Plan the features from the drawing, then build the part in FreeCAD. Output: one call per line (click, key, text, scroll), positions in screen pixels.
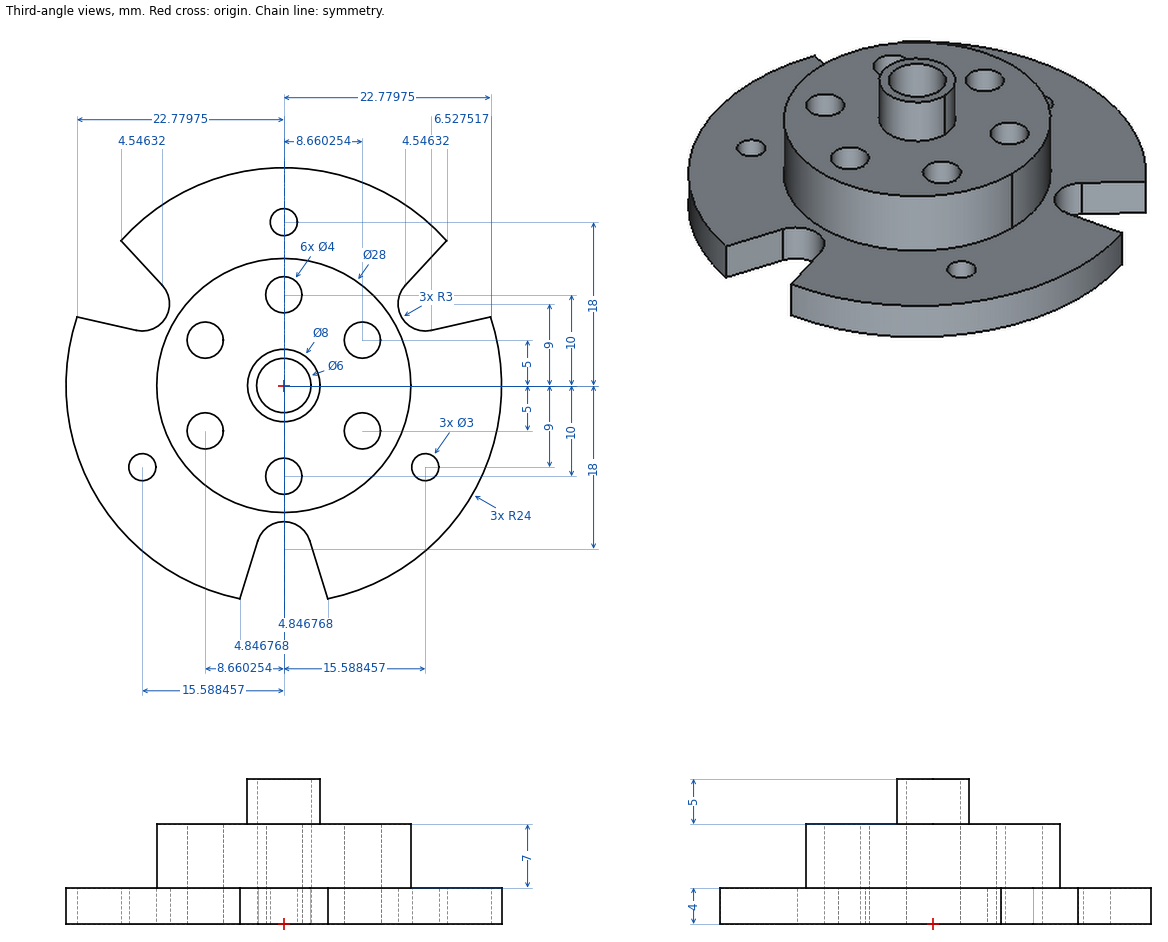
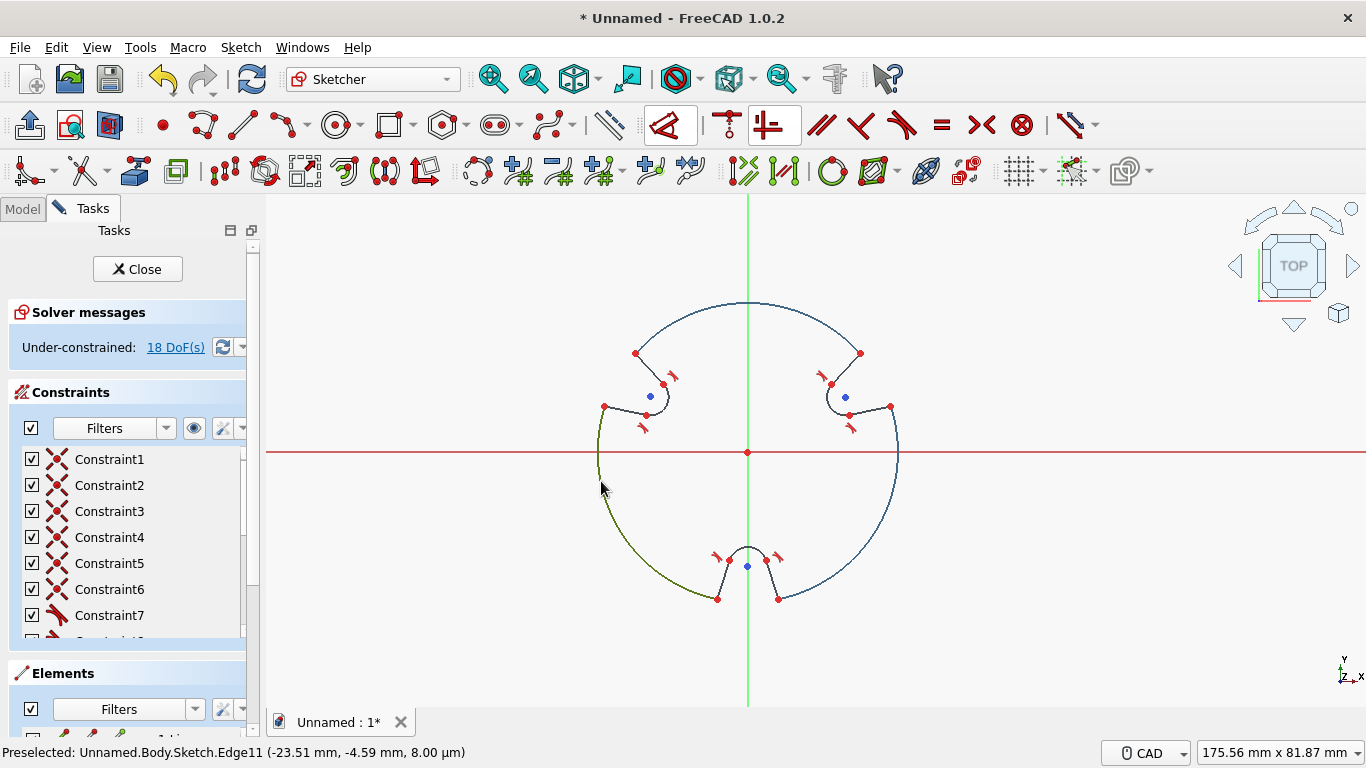
key(e)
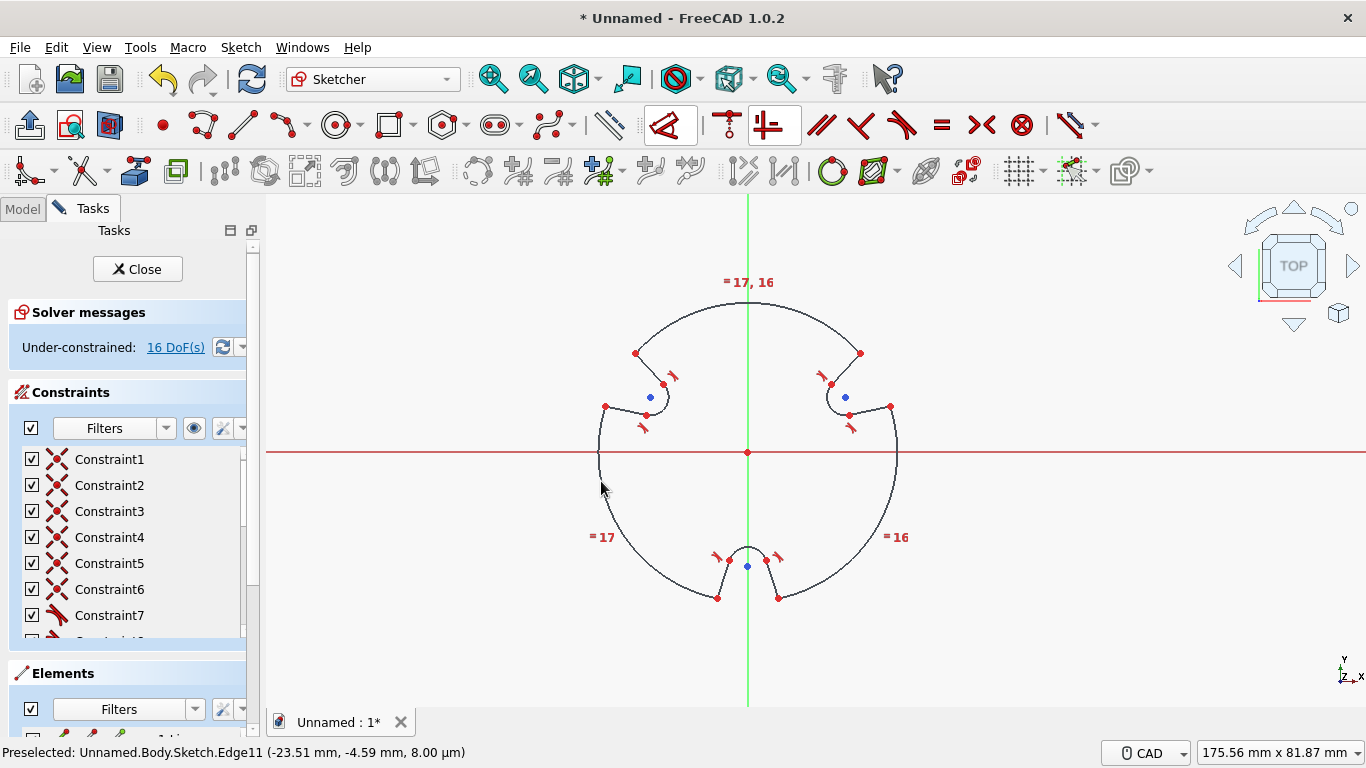
click(827, 397)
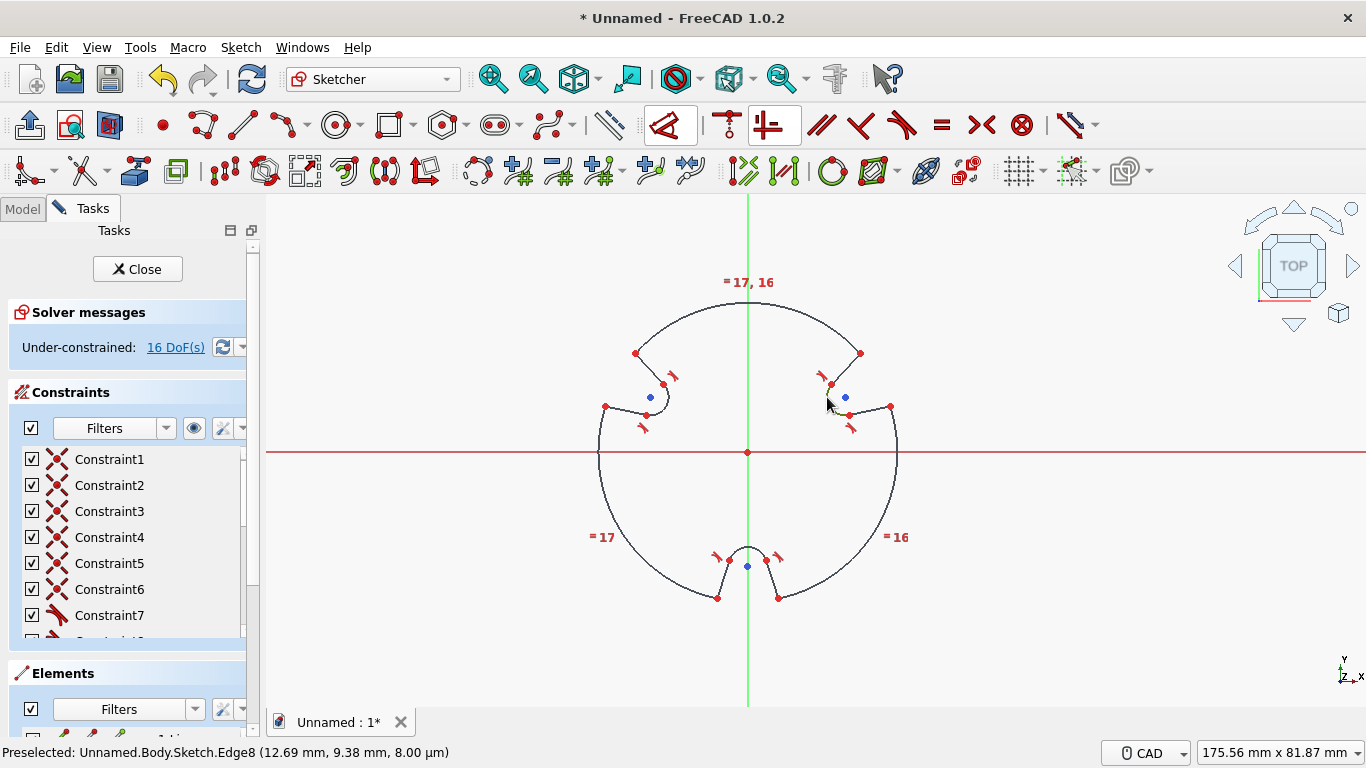
click(660, 413)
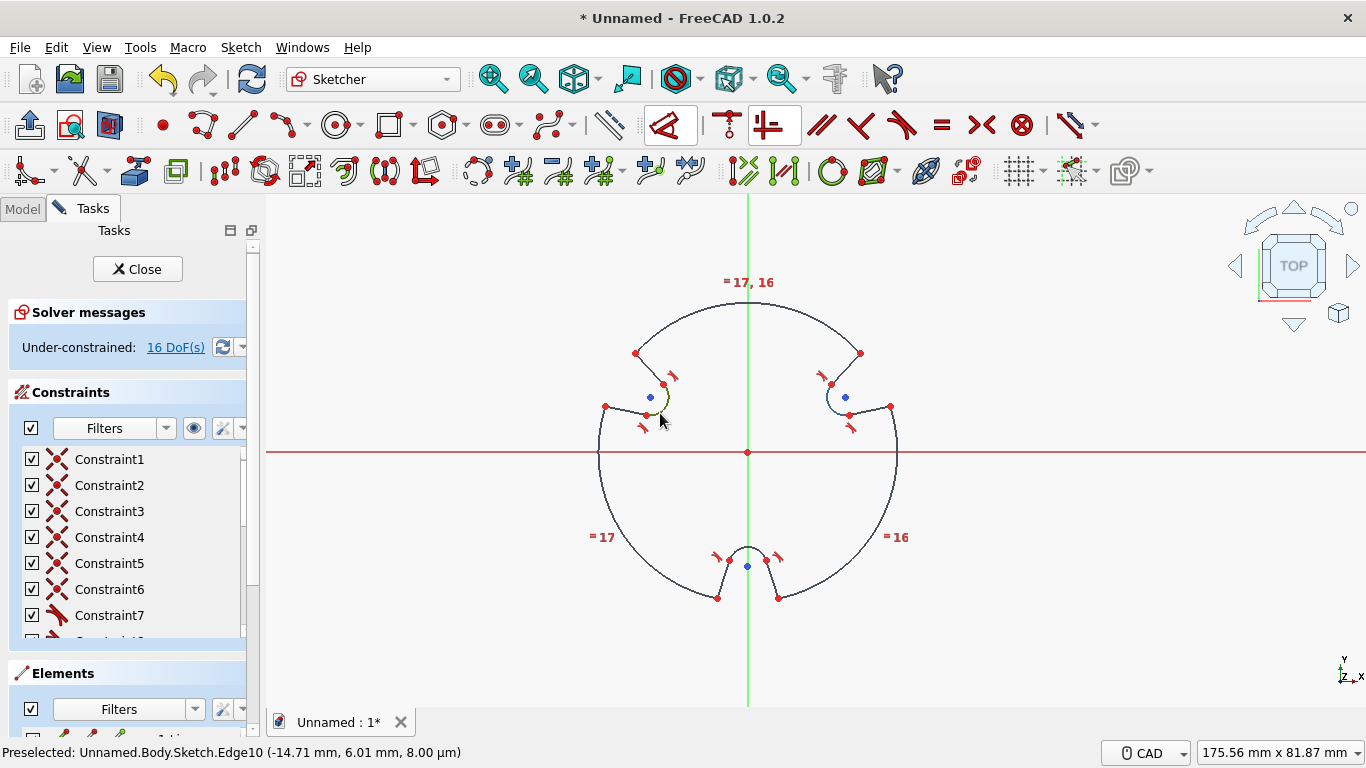
scroll(757, 549, up, 2)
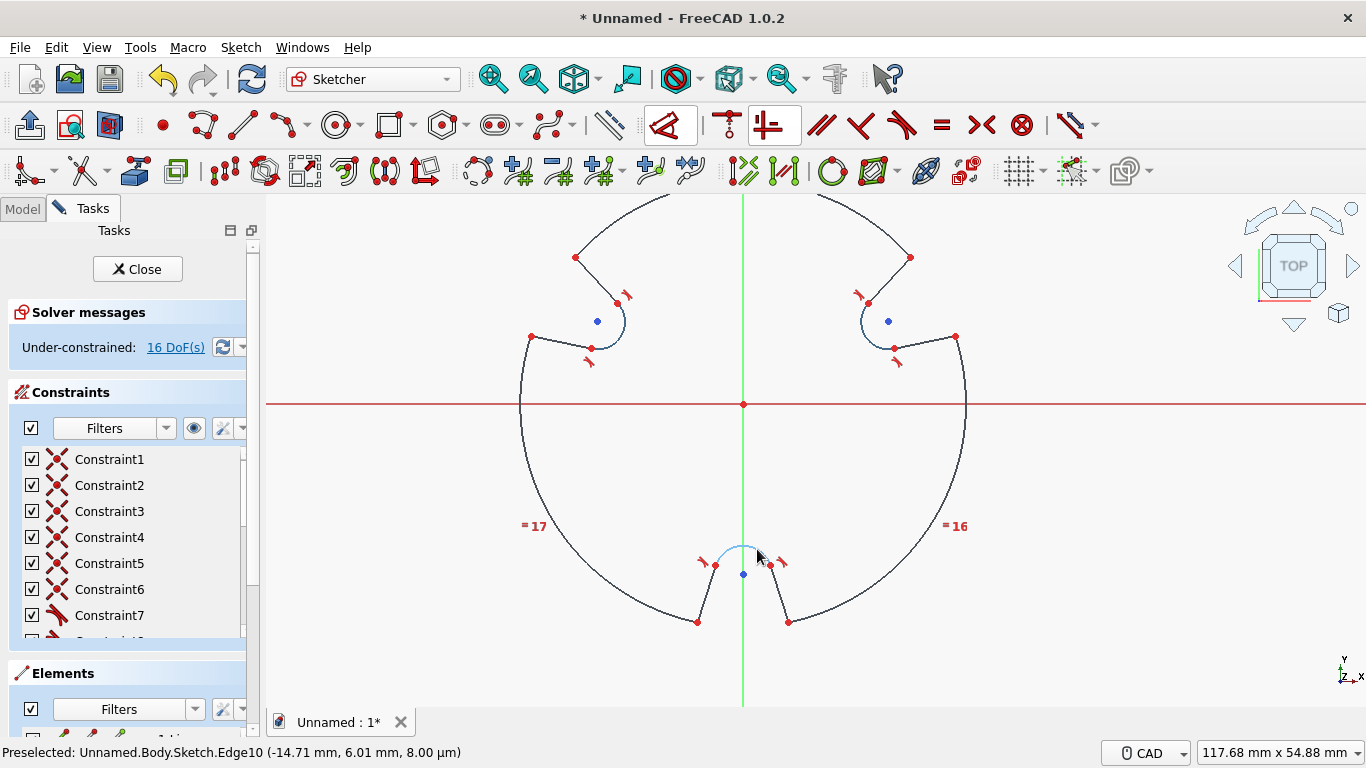
click(757, 549)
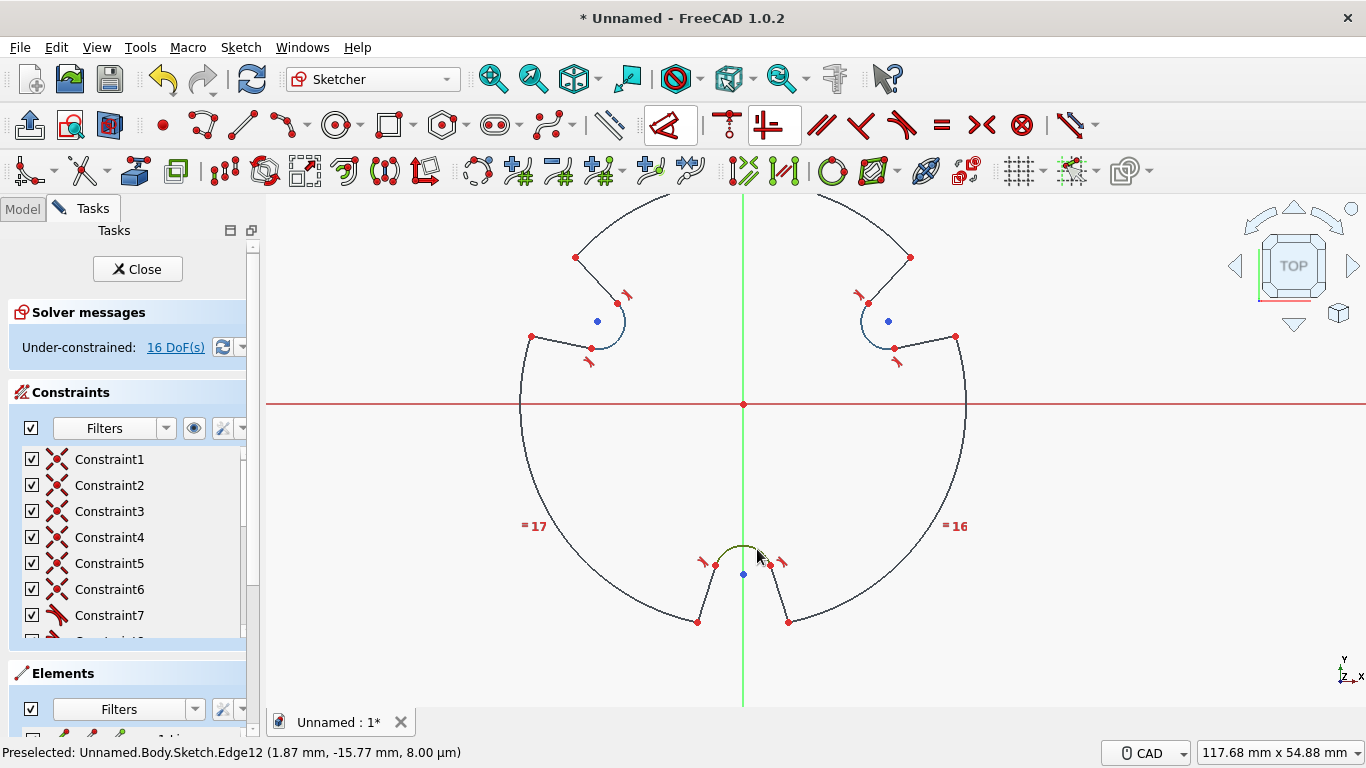
key(e)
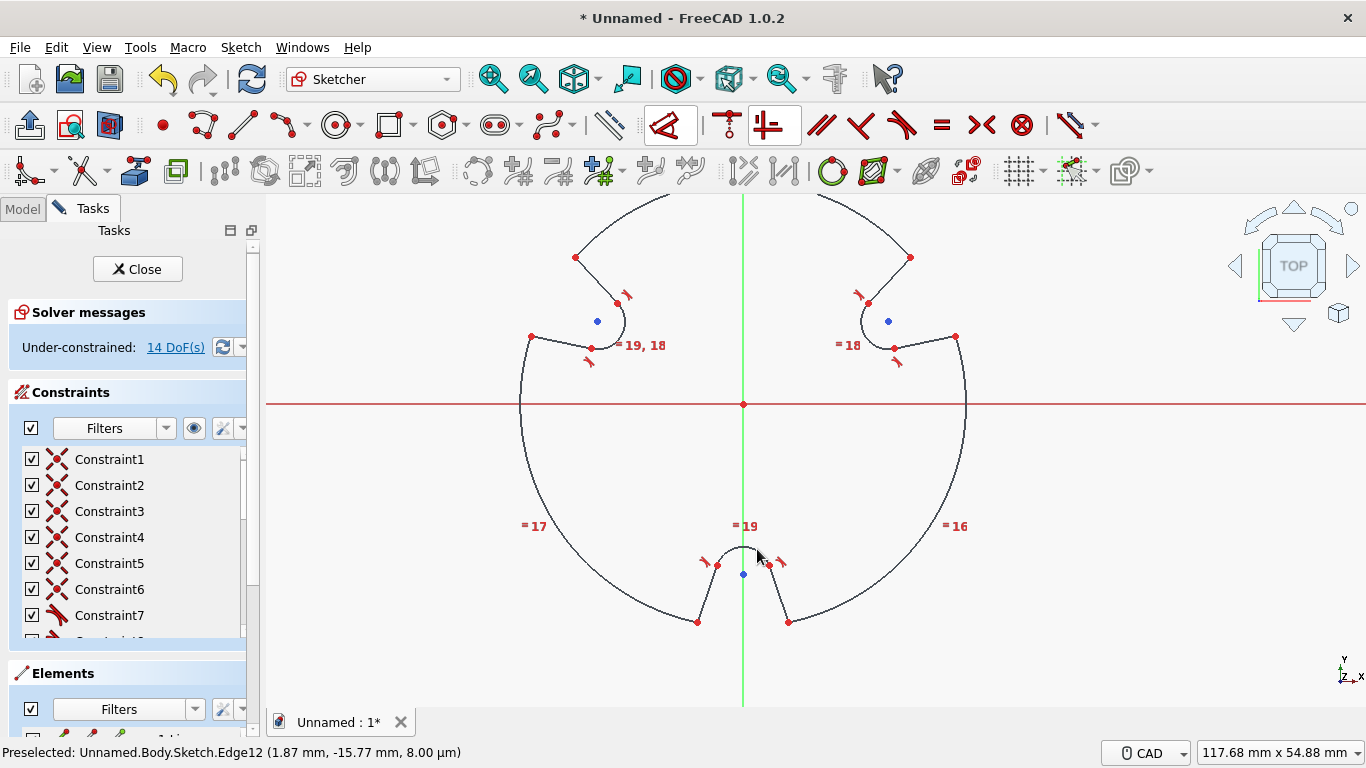
click(743, 574)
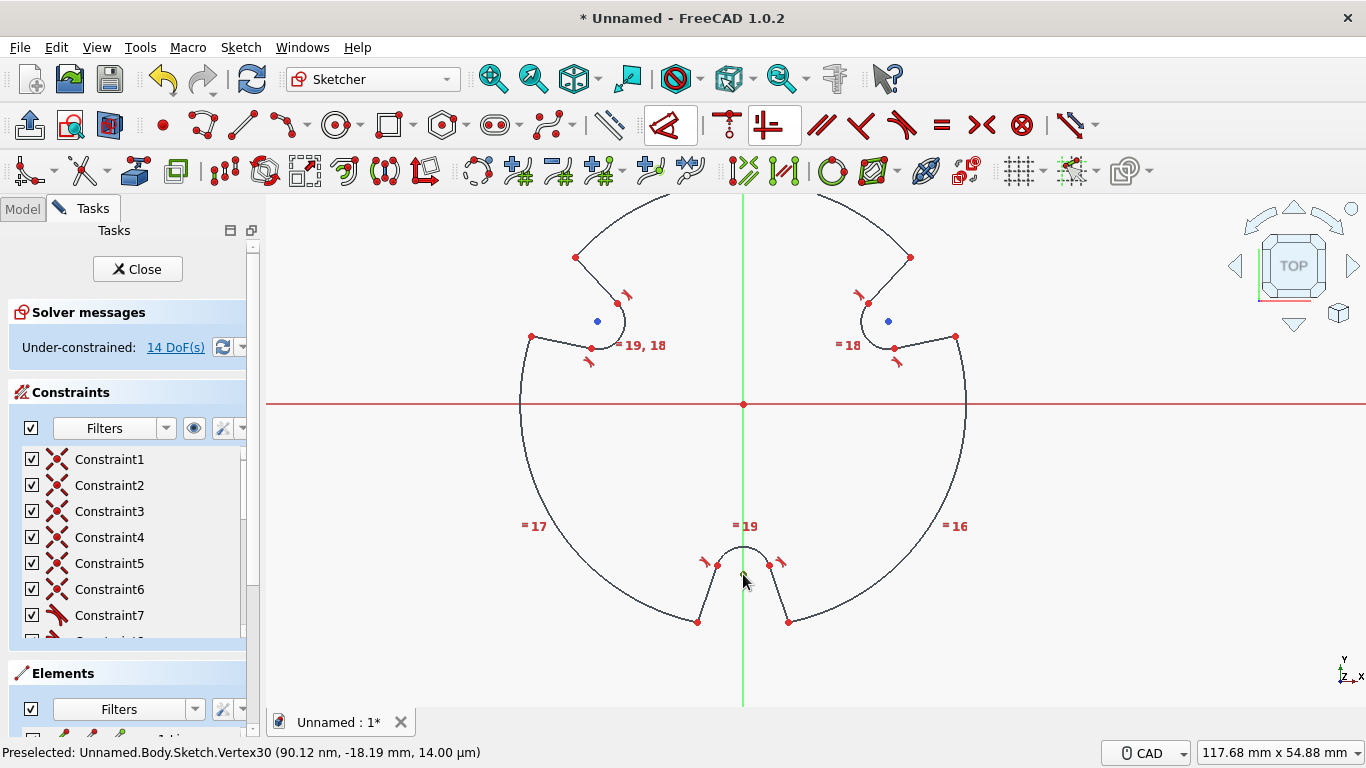
click(743, 646)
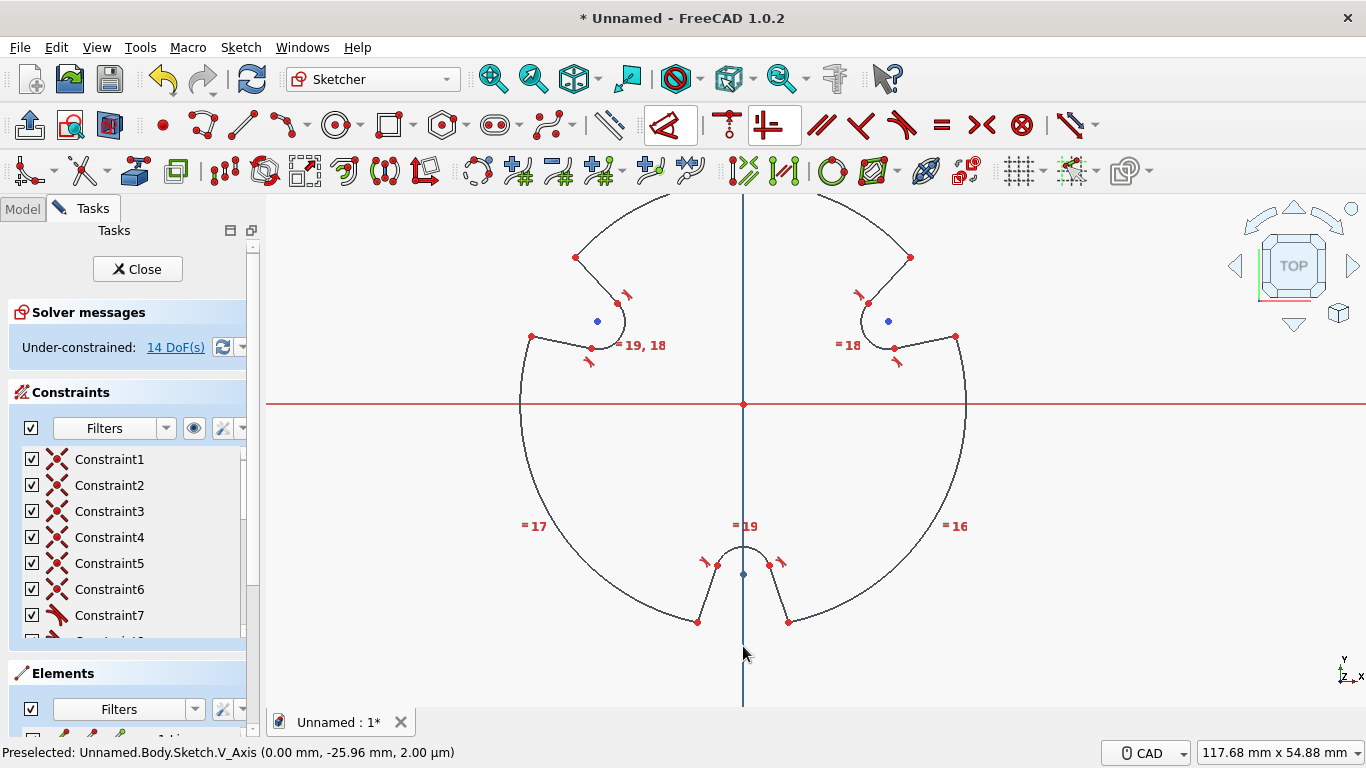
click(728, 126)